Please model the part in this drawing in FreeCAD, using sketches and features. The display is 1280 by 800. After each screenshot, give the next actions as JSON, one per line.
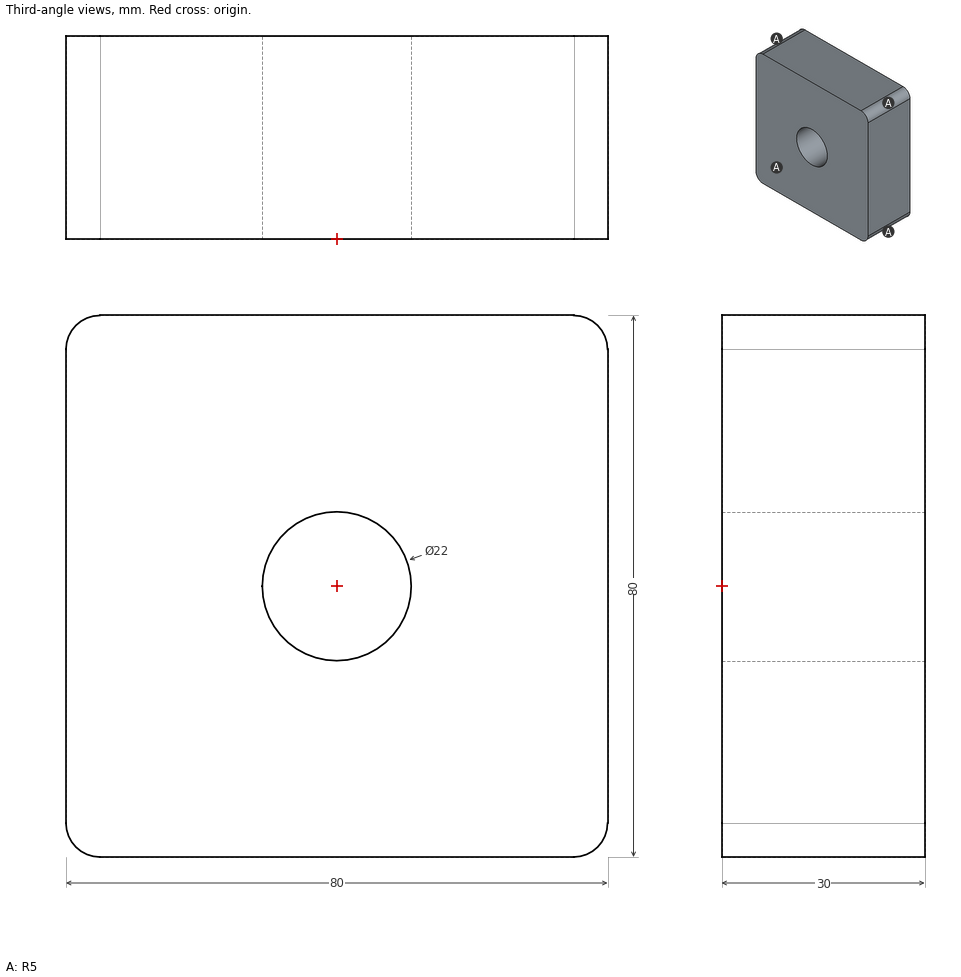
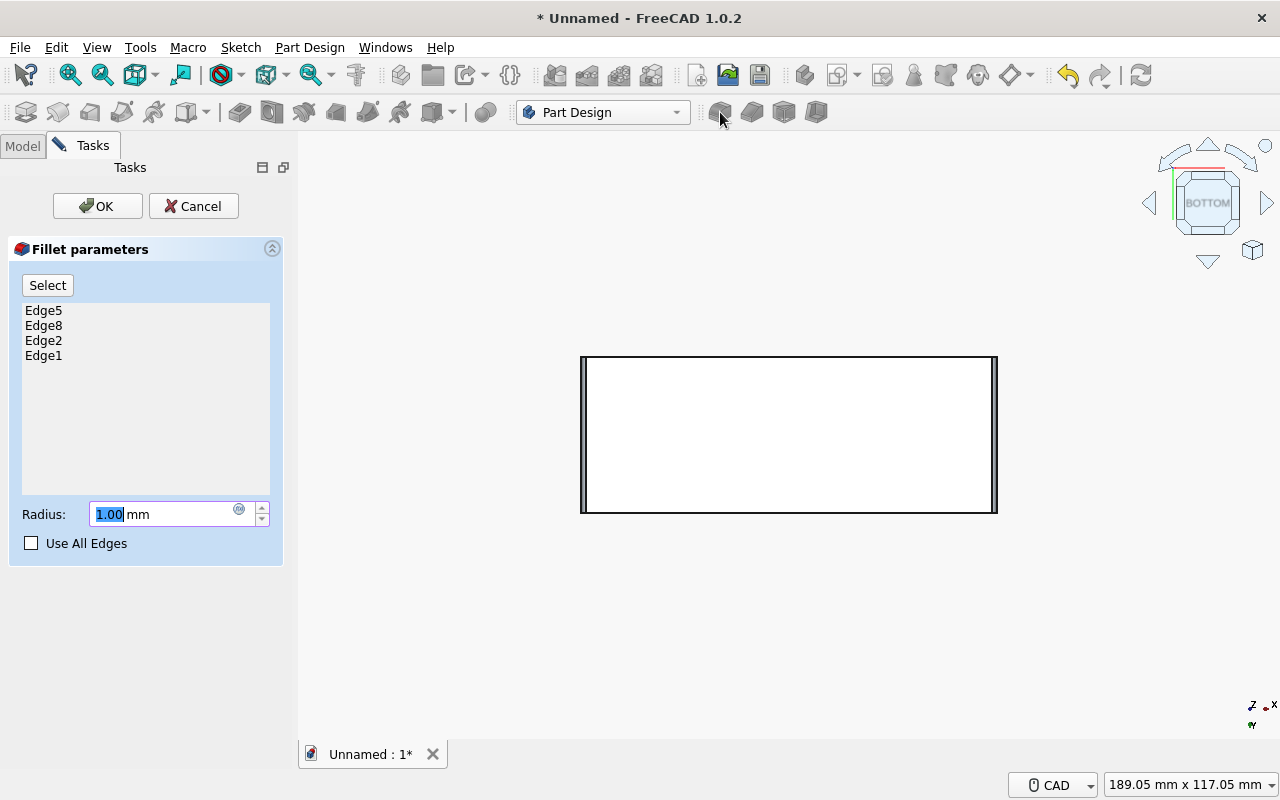
{"action": "type", "text": "5"}
{"action": "key", "text": "Tab"}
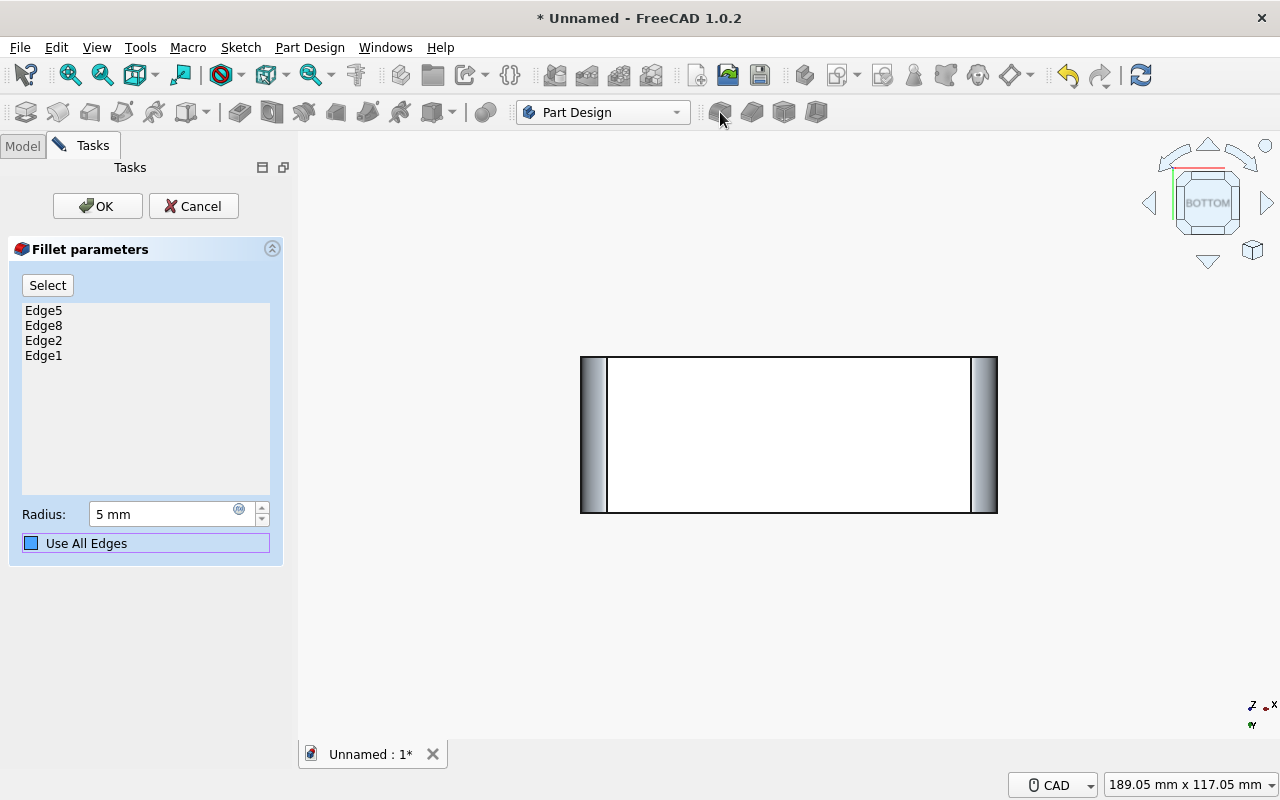
{"action": "left_click", "coordinate": [98, 206]}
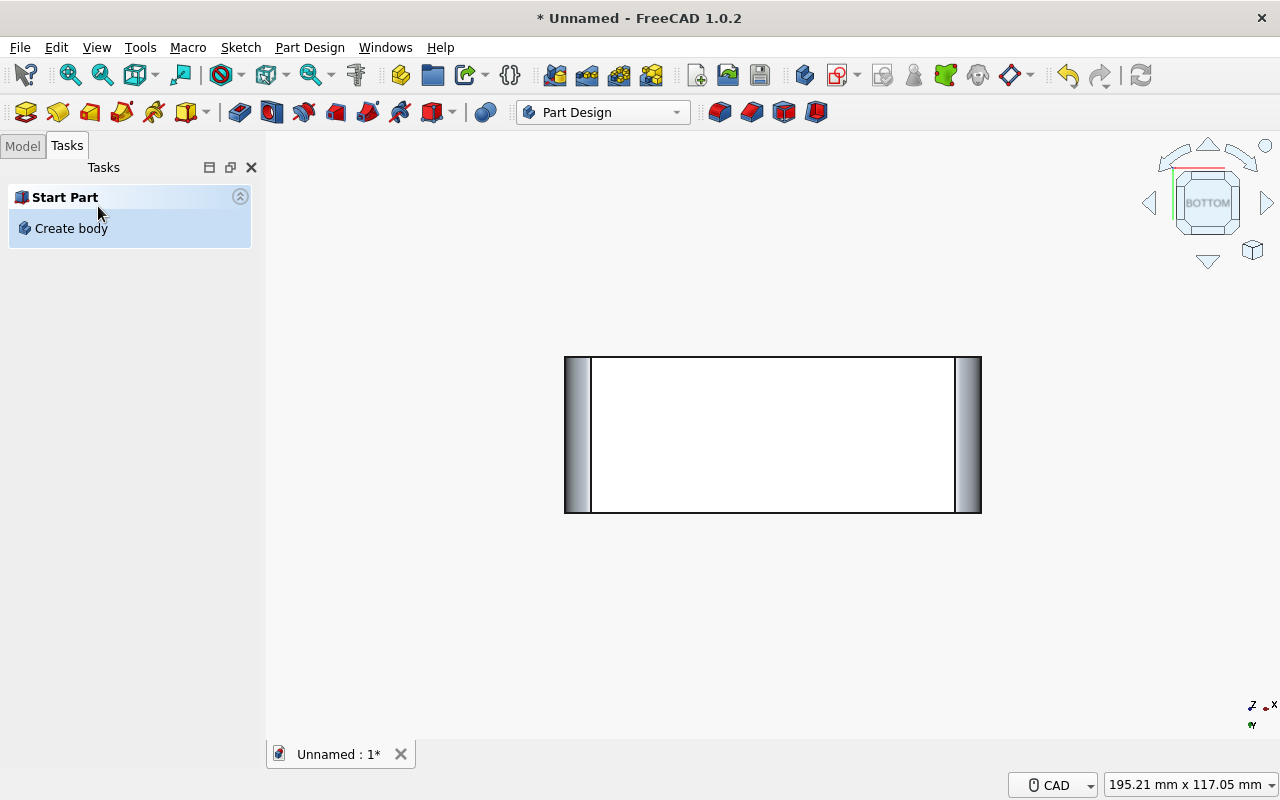
{"action": "left_click", "coordinate": [72, 76]}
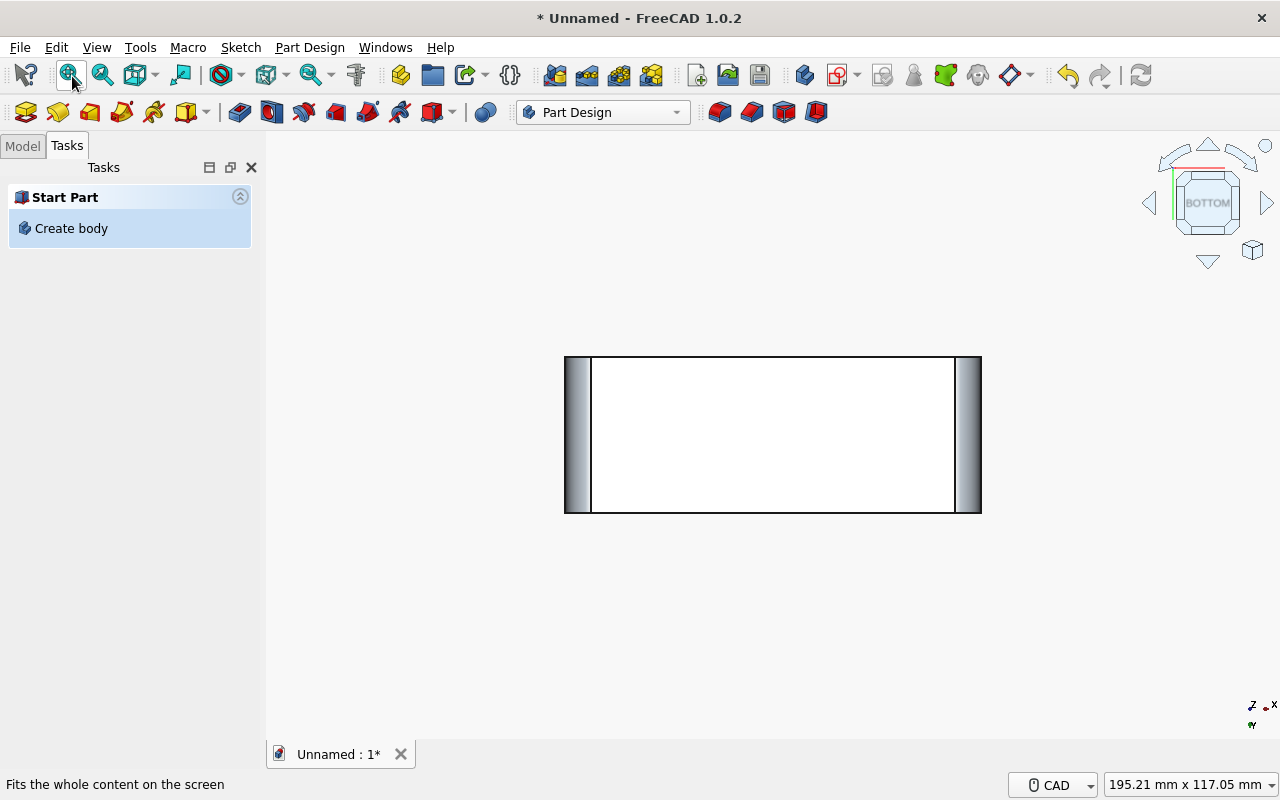
{"action": "key", "text": "4"}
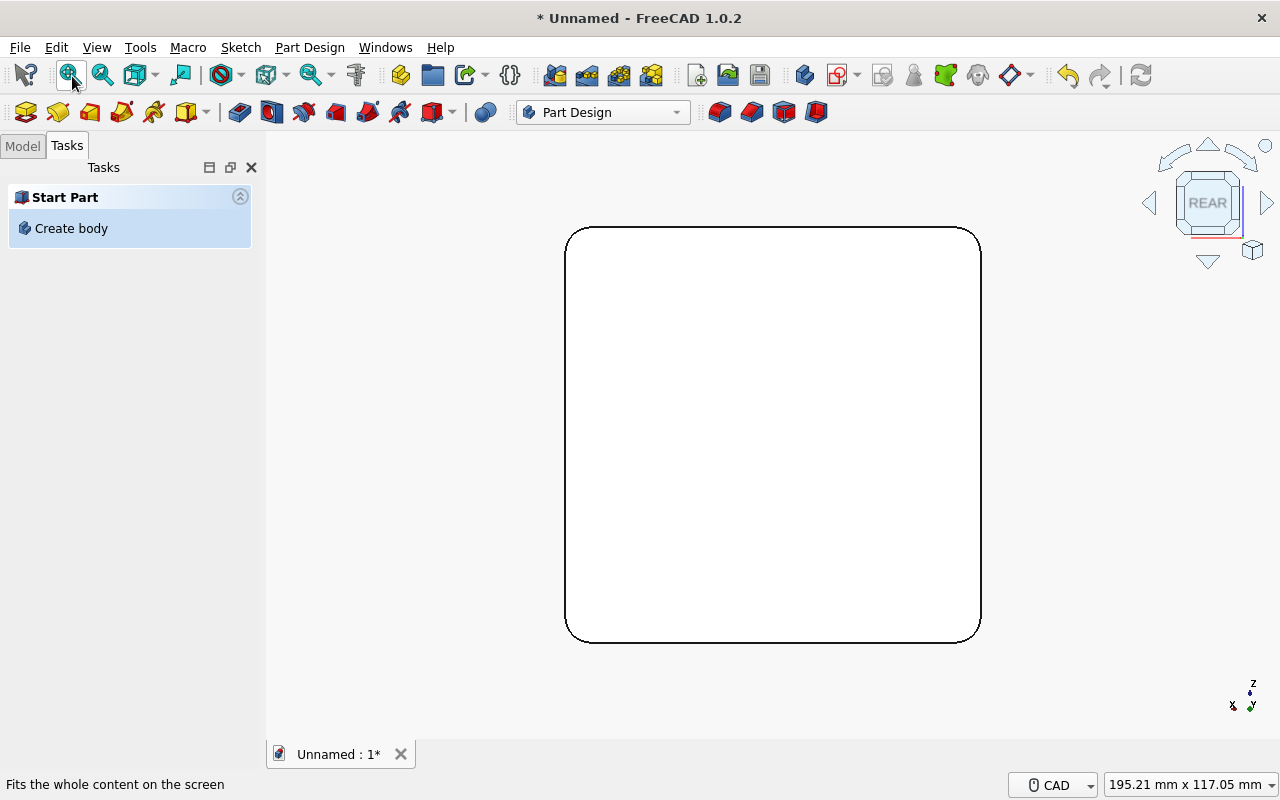
{"action": "left_click", "coordinate": [773, 434]}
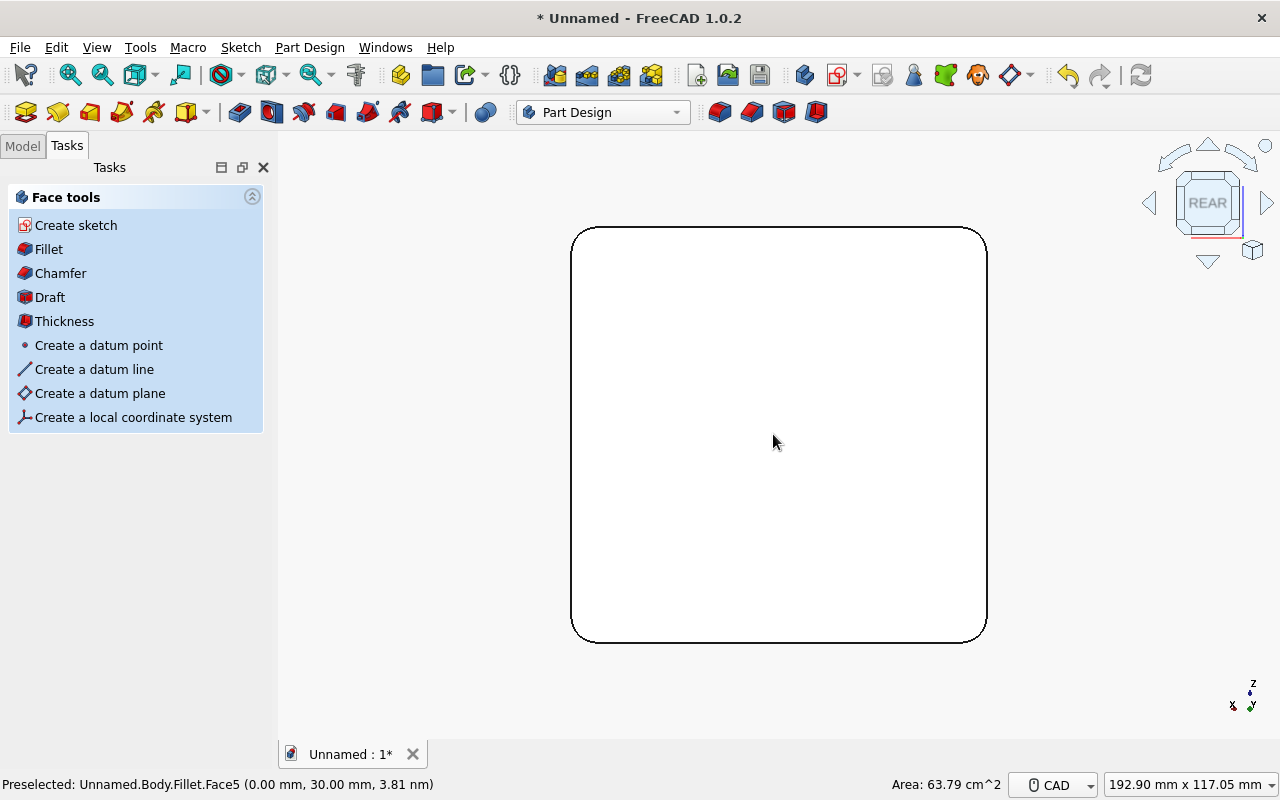
{"action": "left_click", "coordinate": [838, 76]}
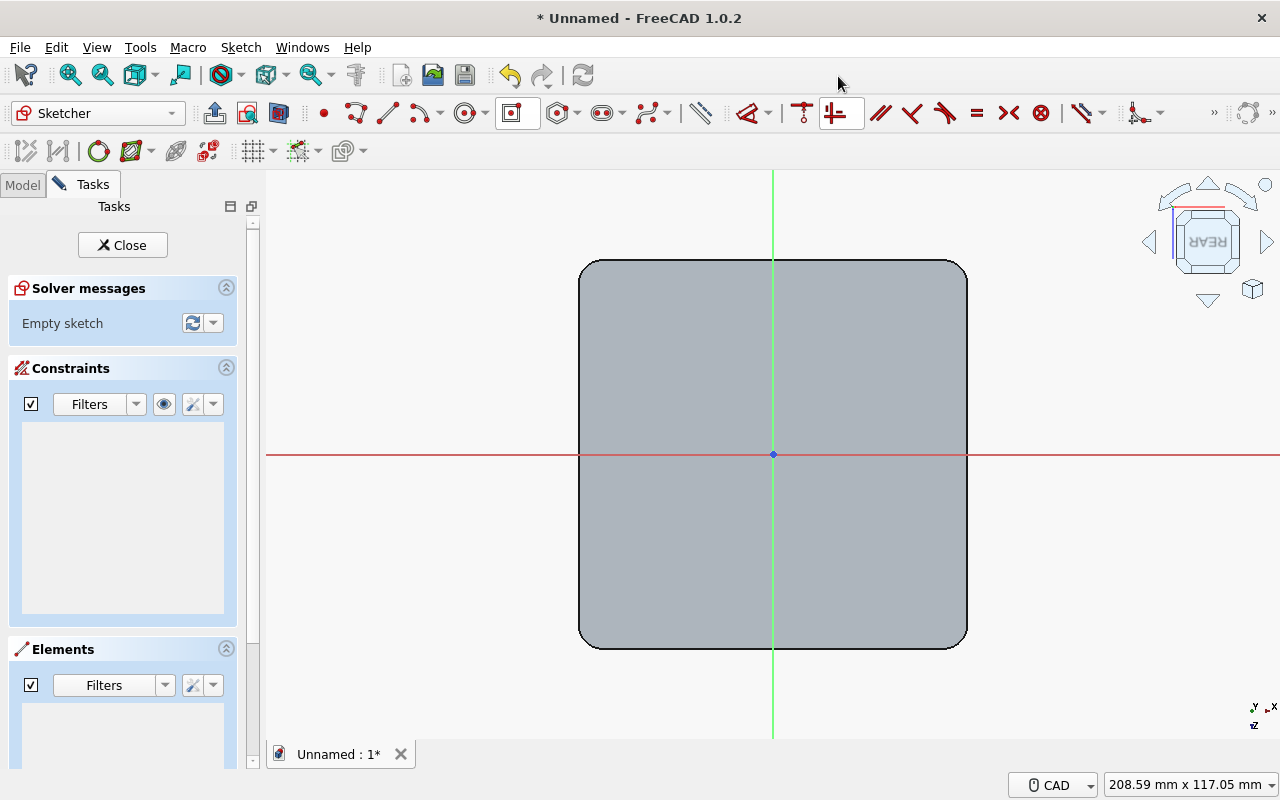
{"action": "scroll", "coordinate": [803, 454], "scroll_direction": "up", "scroll_amount": 6}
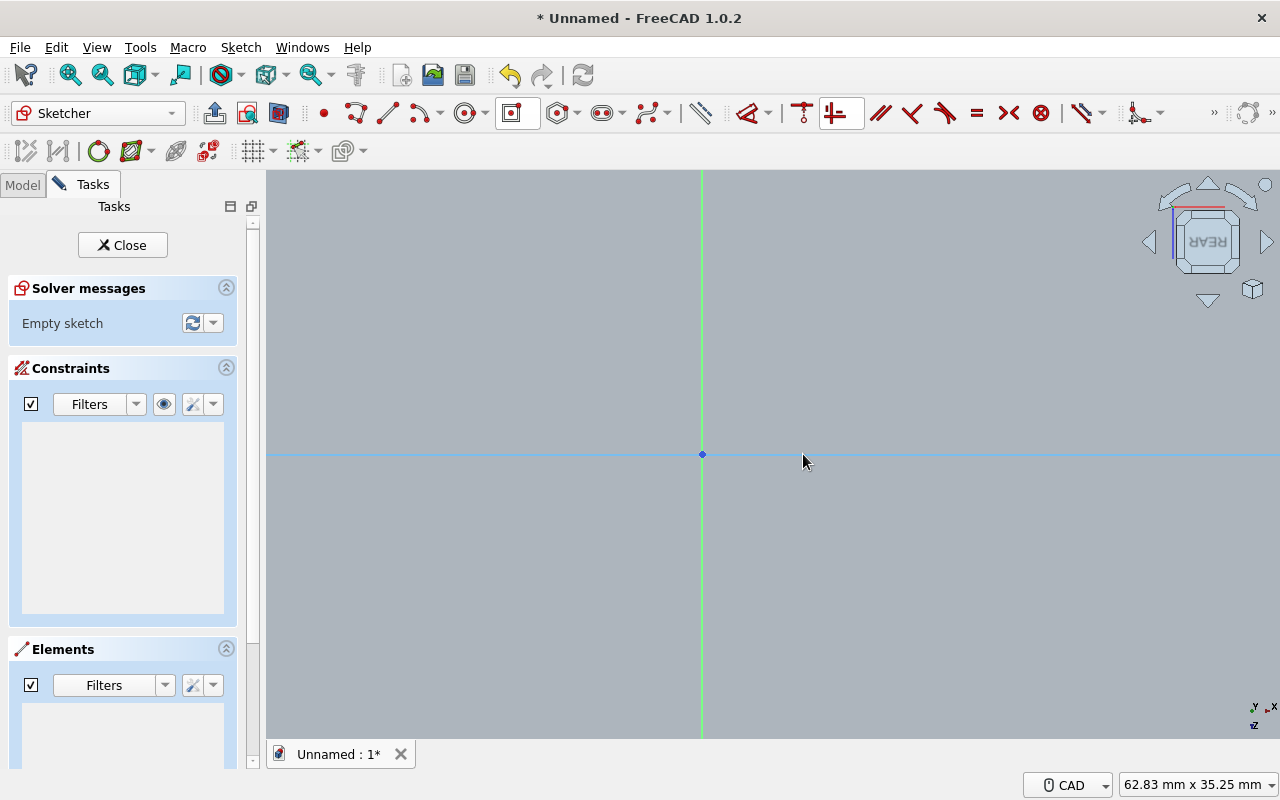
{"action": "left_click", "coordinate": [466, 114]}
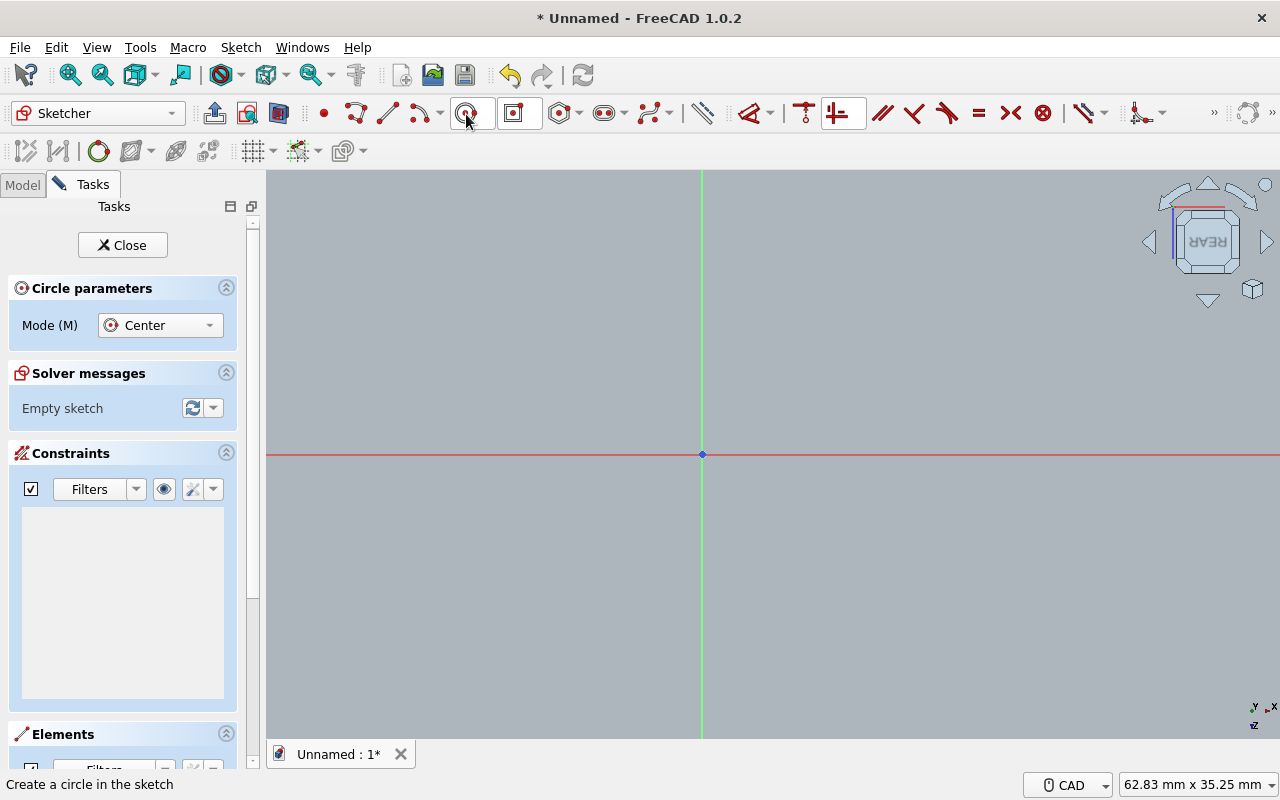
{"action": "left_click", "coordinate": [702, 454]}
{"action": "left_click", "coordinate": [828, 329]}
{"action": "key", "text": "Escape"}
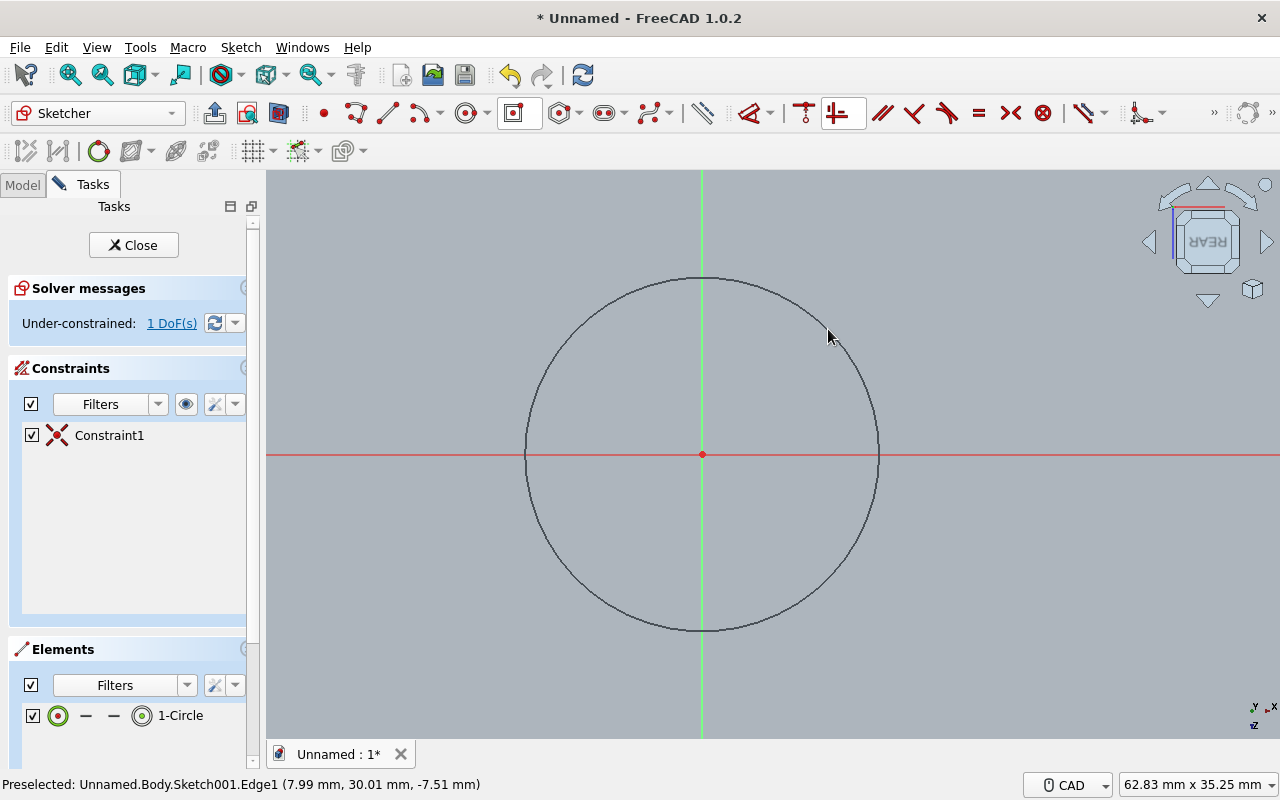
{"action": "left_click", "coordinate": [750, 114]}